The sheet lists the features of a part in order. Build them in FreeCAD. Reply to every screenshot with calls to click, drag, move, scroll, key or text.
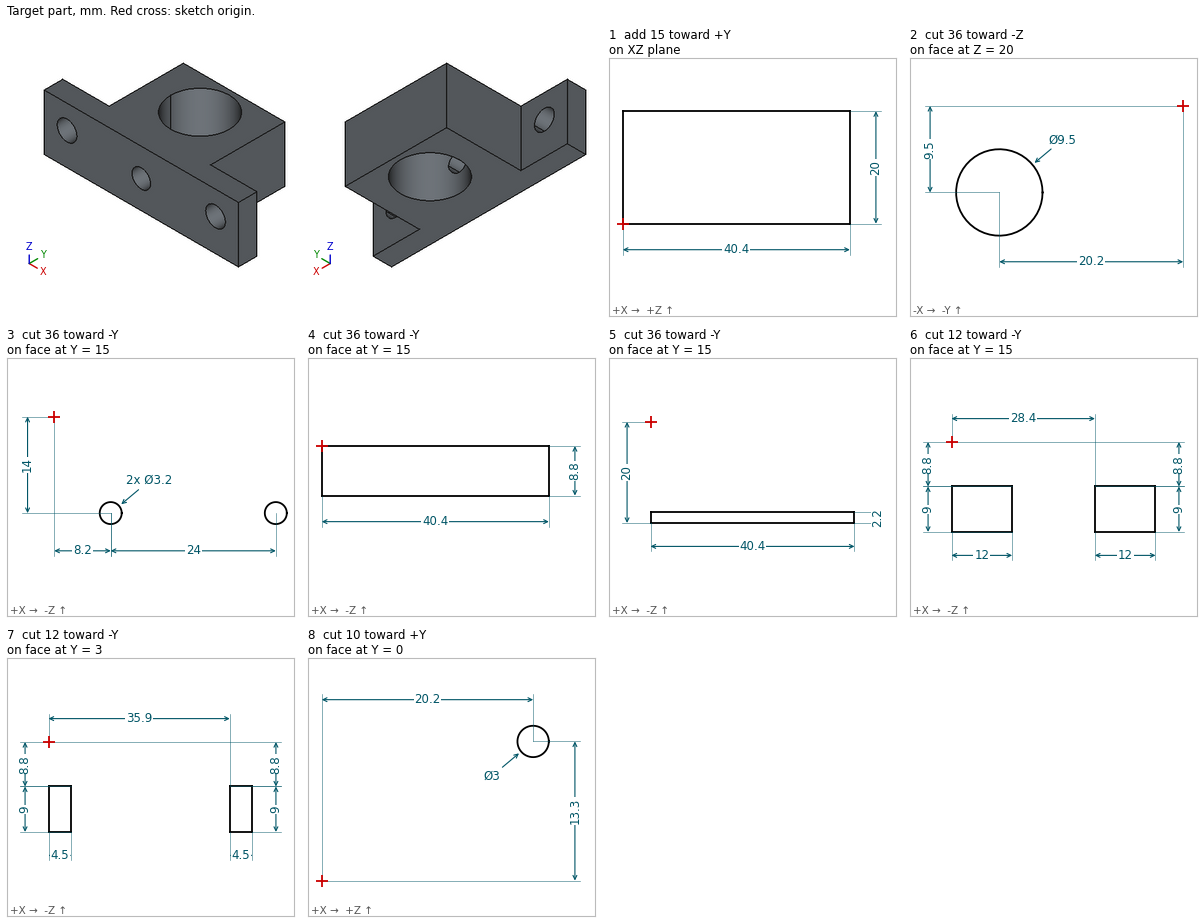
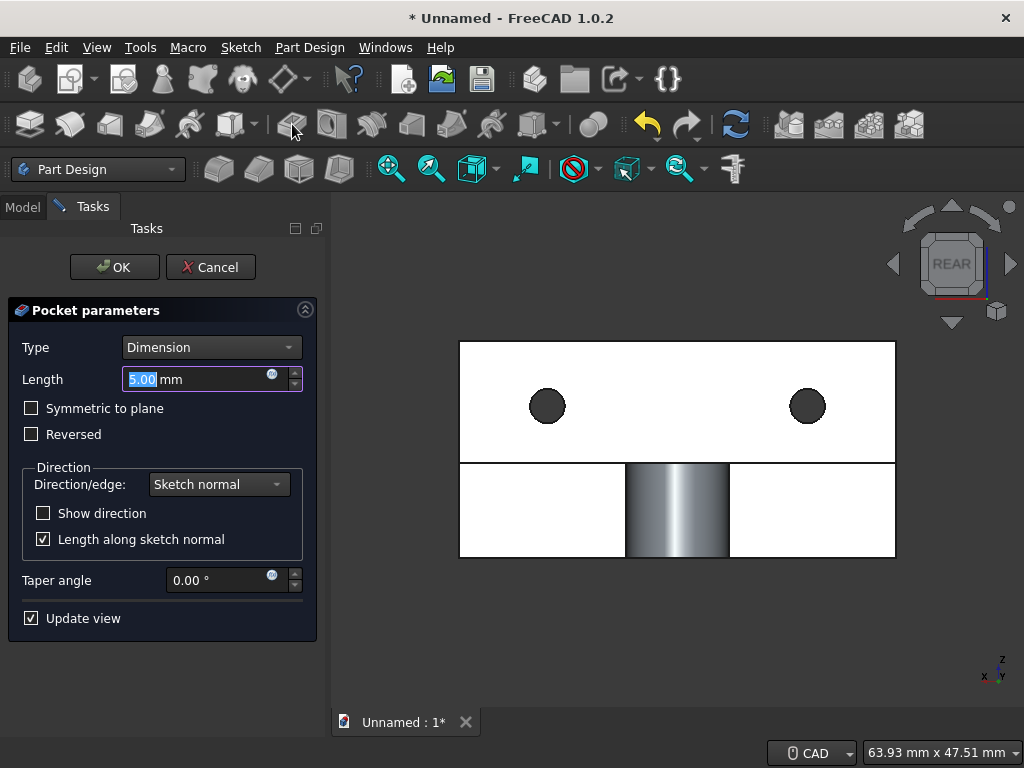
text(36)
key(Tab)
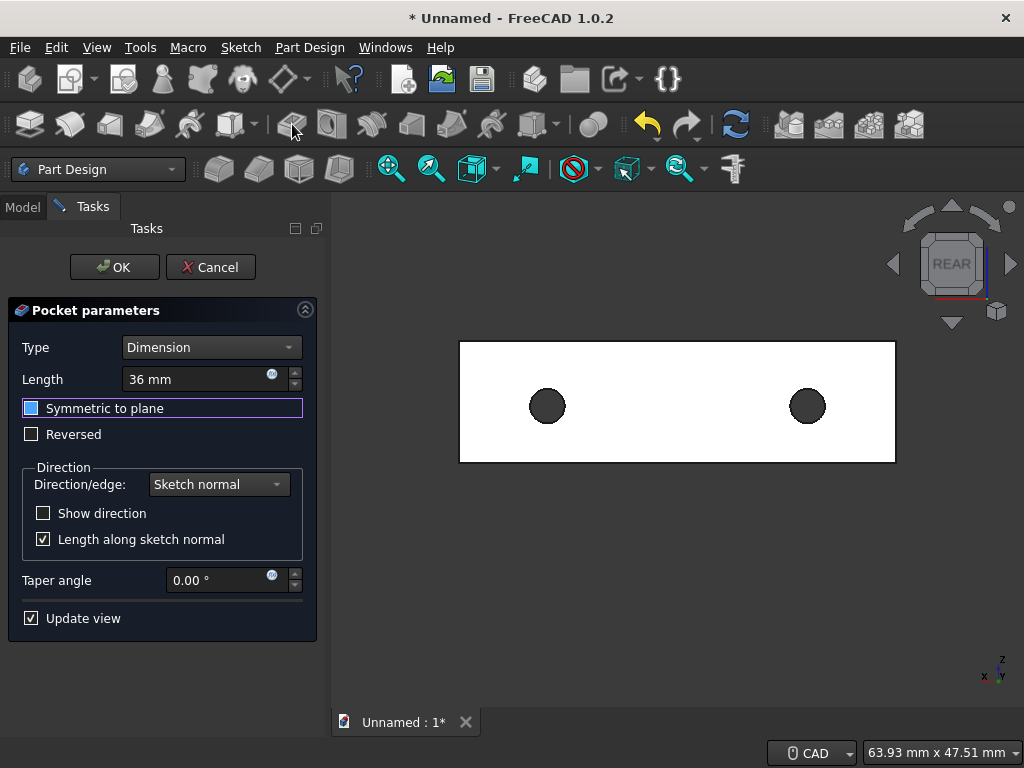
click(115, 267)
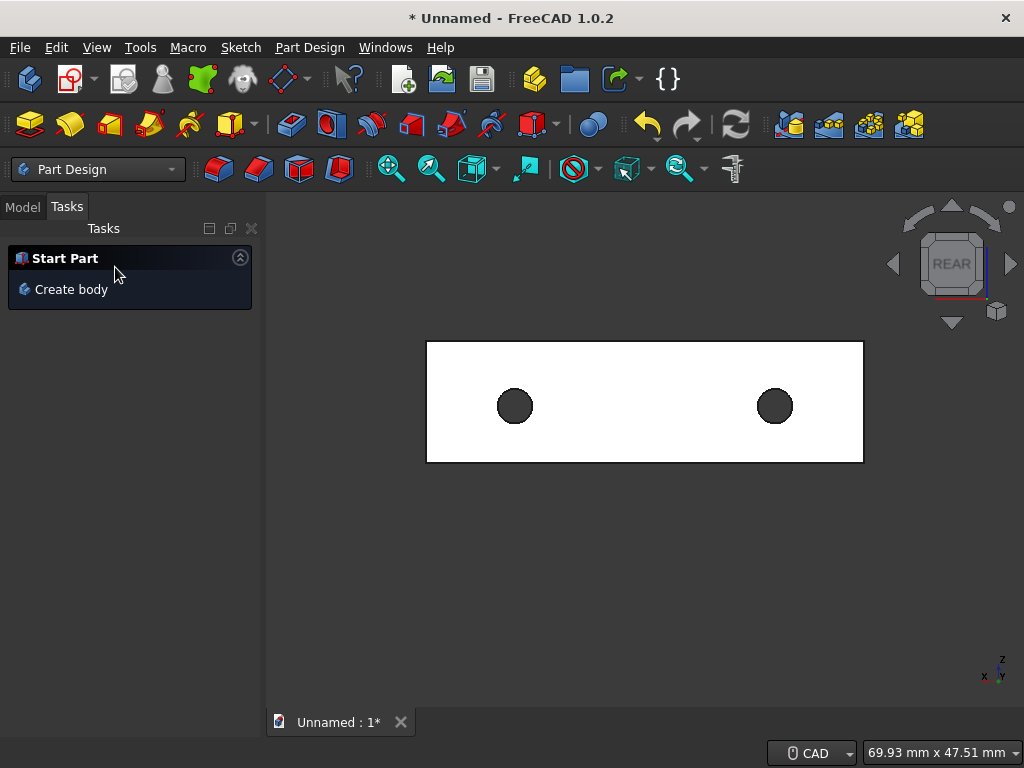
click(645, 401)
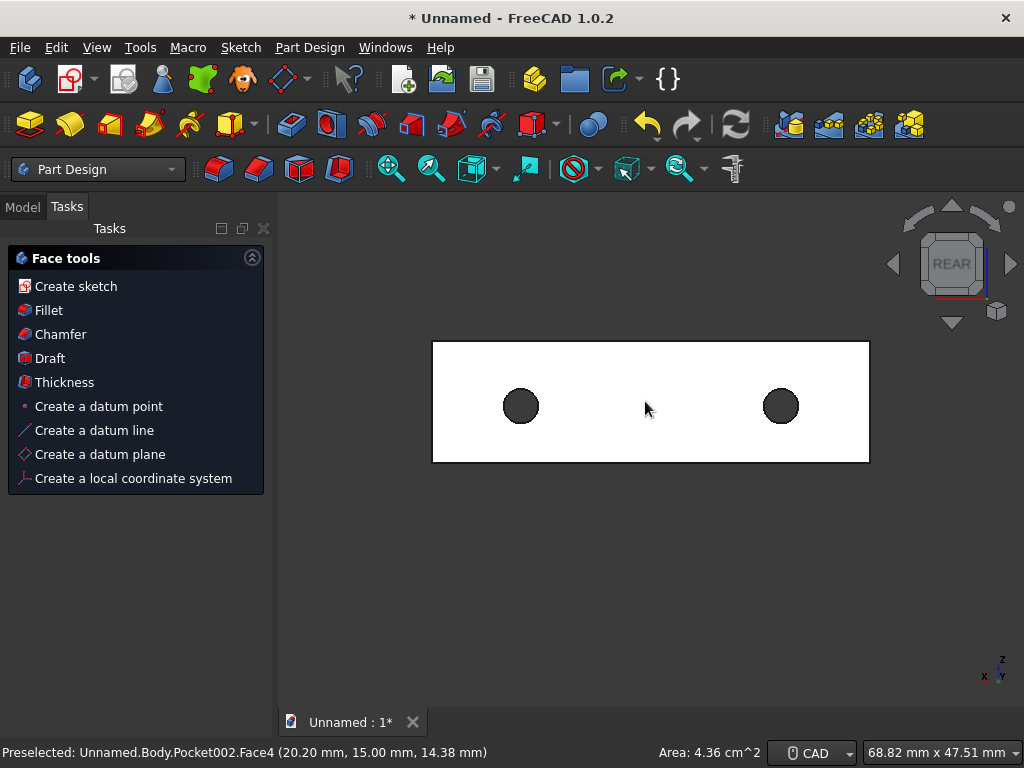
click(70, 80)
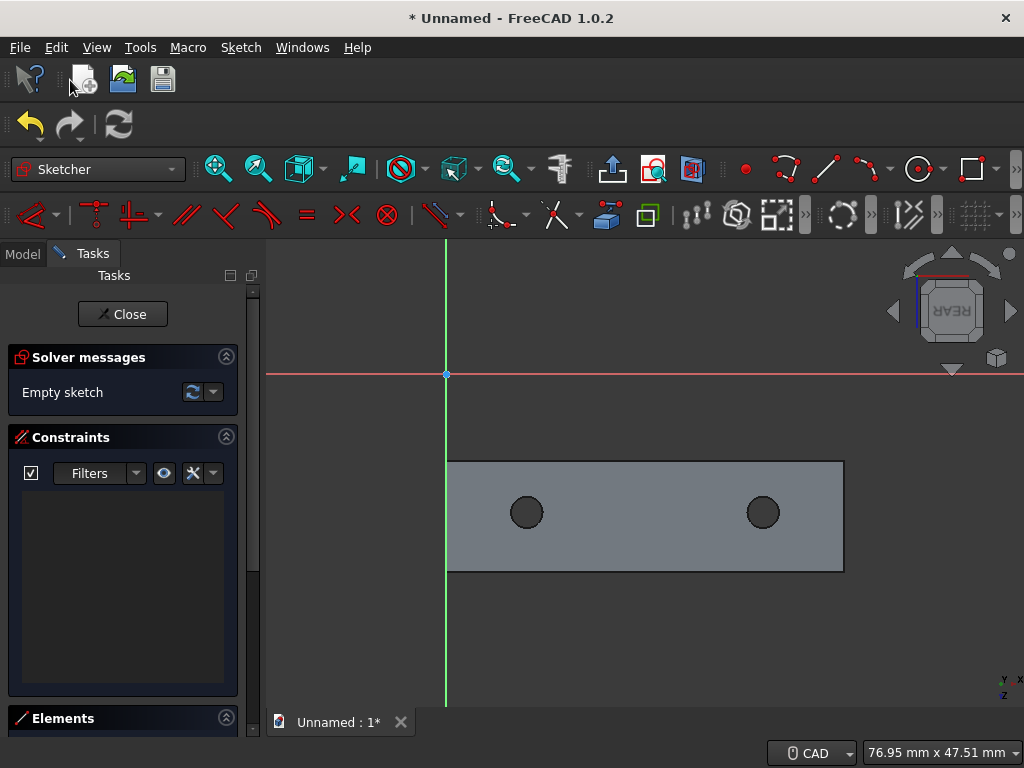
scroll(294, 473, down, 1)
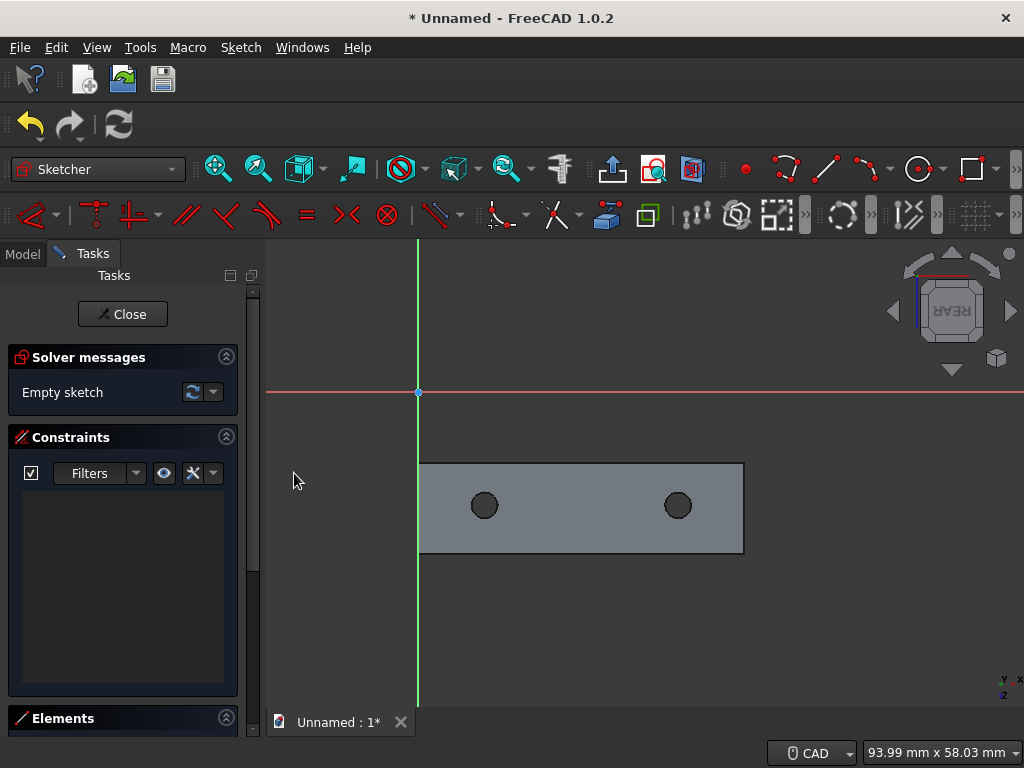
click(972, 170)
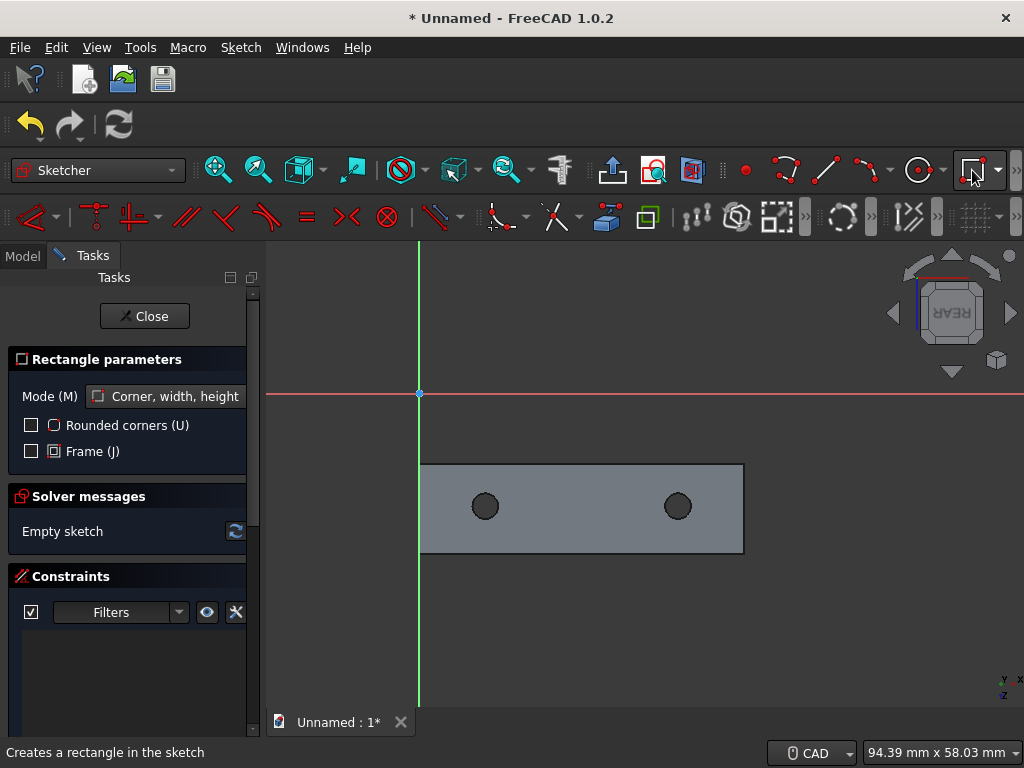
click(419, 537)
move(744, 554)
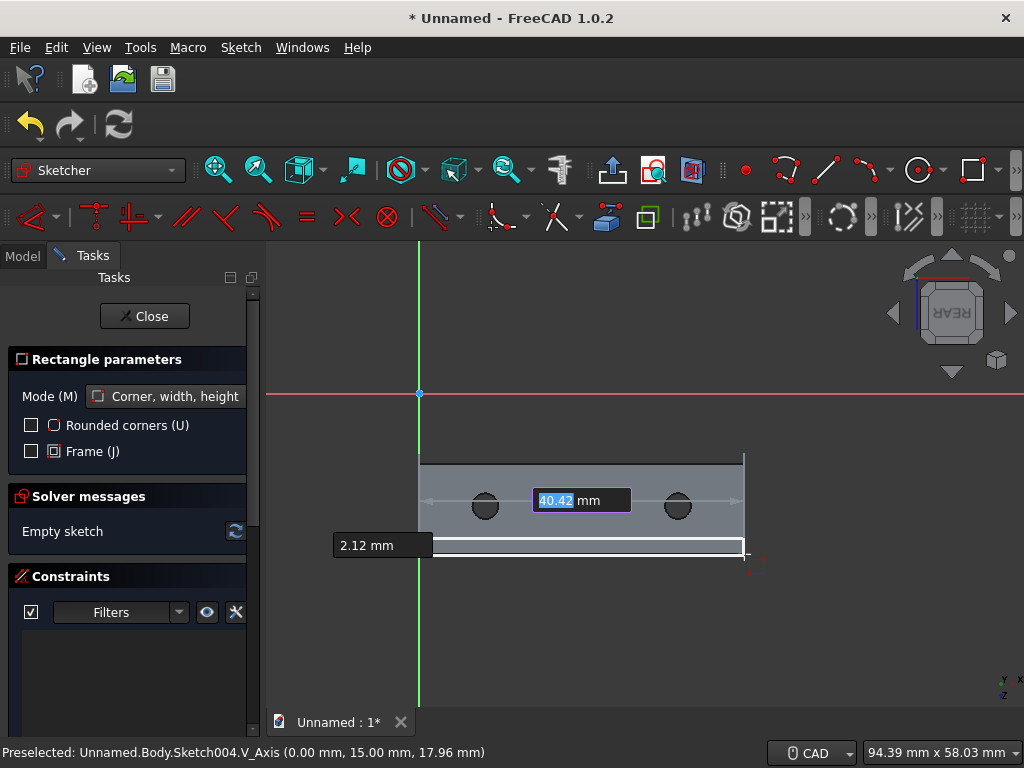
text(40.4)
key(Tab)
text(2.2)
key(Return)
key(Escape)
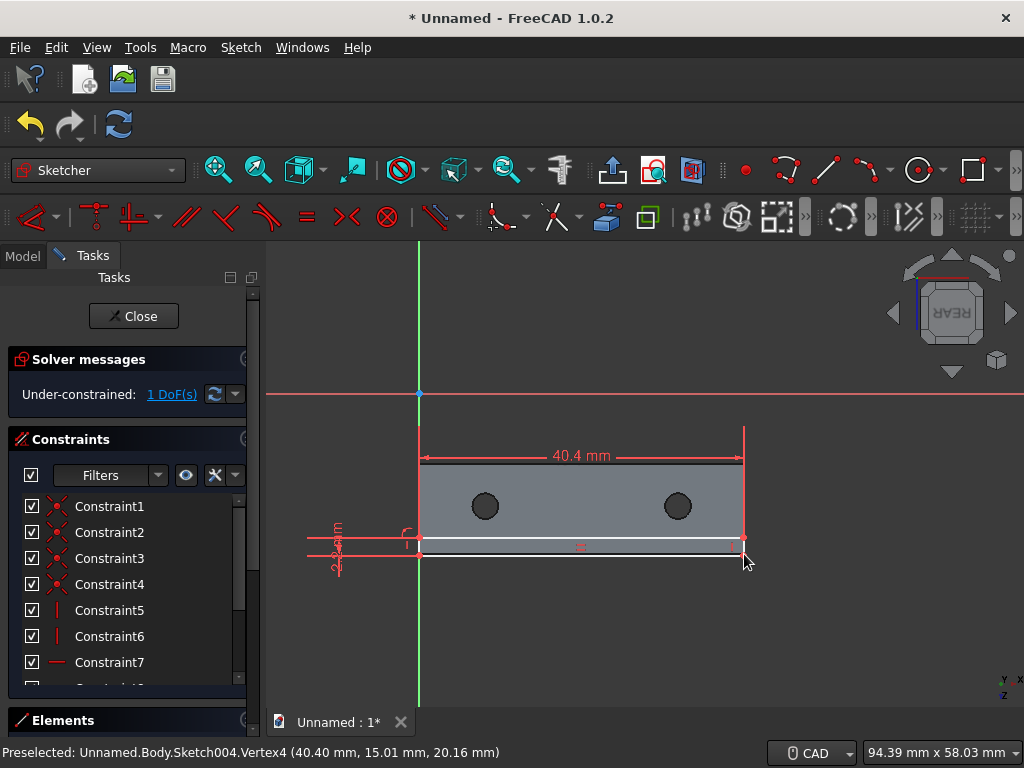
click(419, 556)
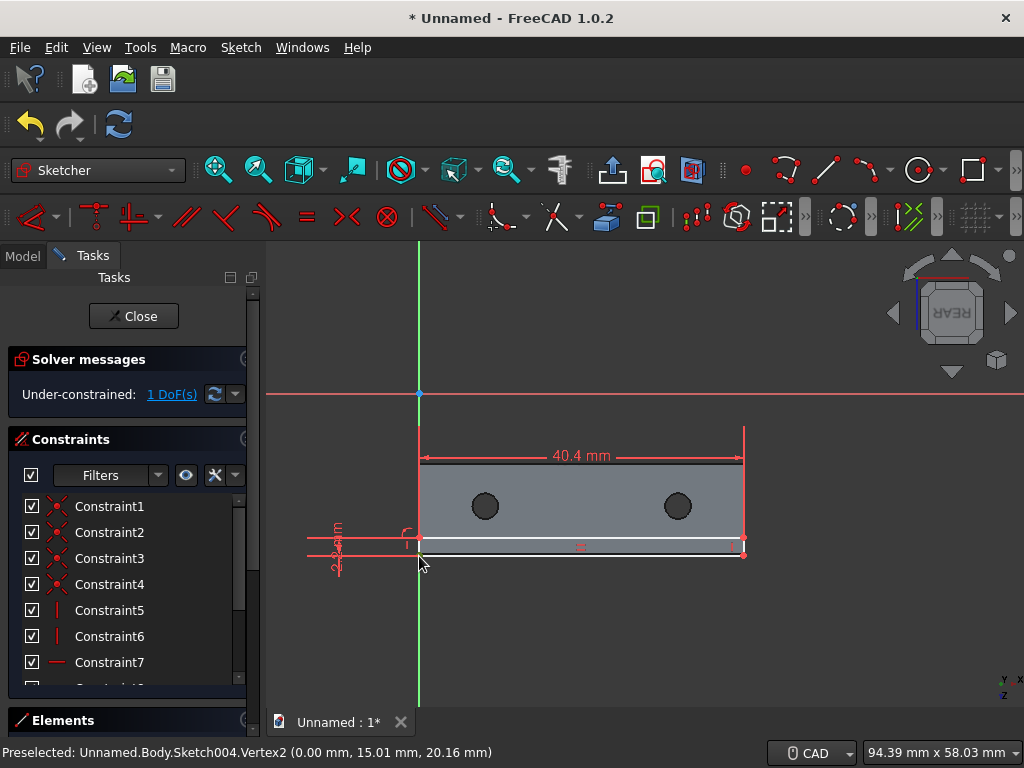
key(i)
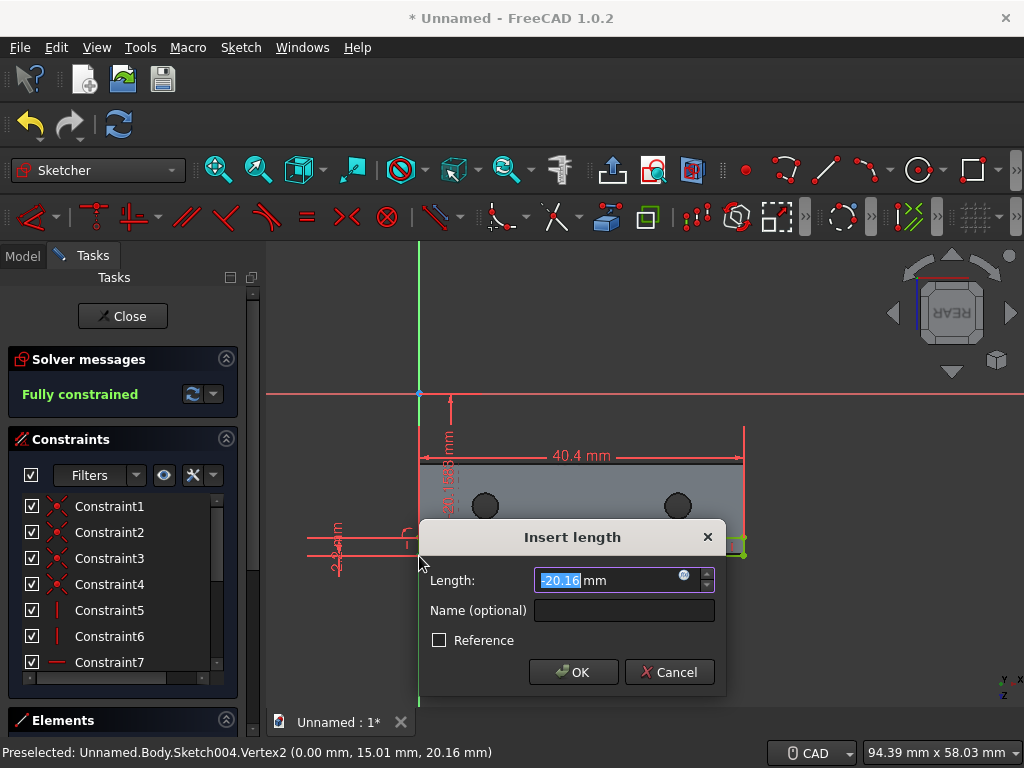
text(-20)
key(Return)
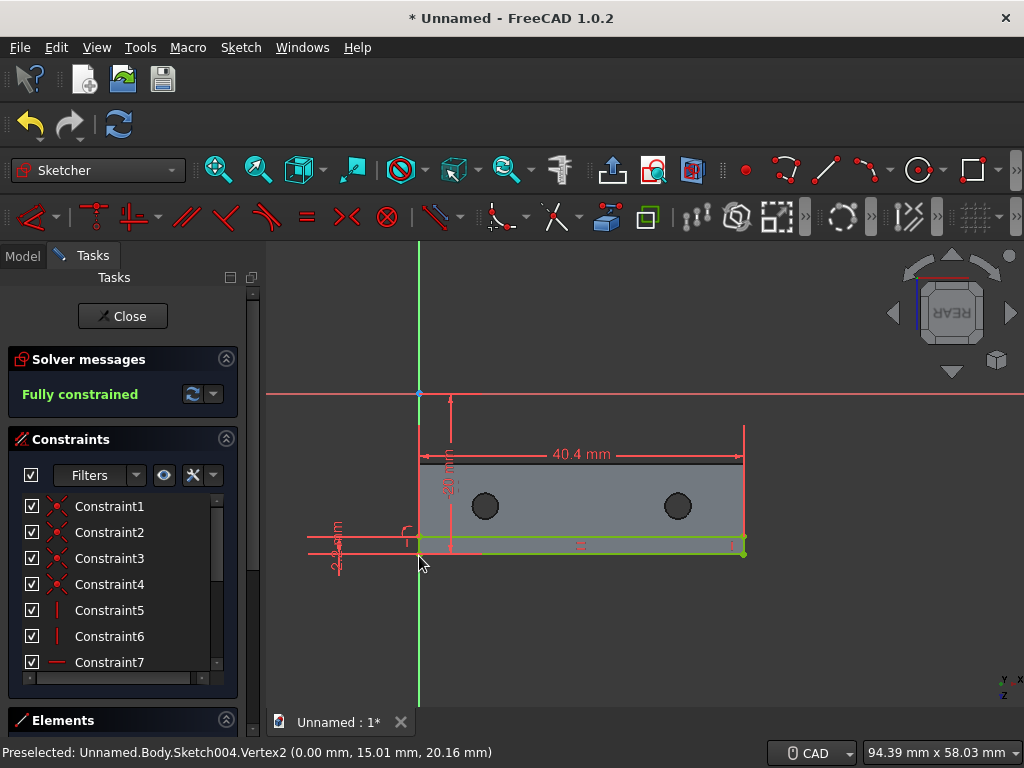
click(123, 316)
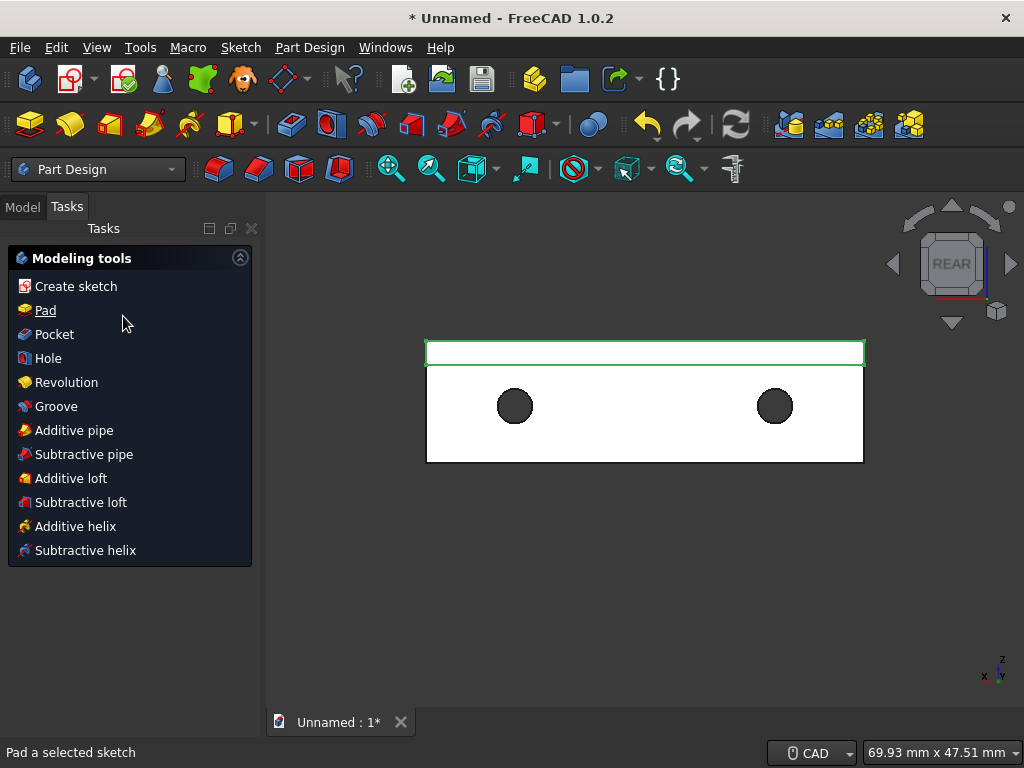
click(292, 124)